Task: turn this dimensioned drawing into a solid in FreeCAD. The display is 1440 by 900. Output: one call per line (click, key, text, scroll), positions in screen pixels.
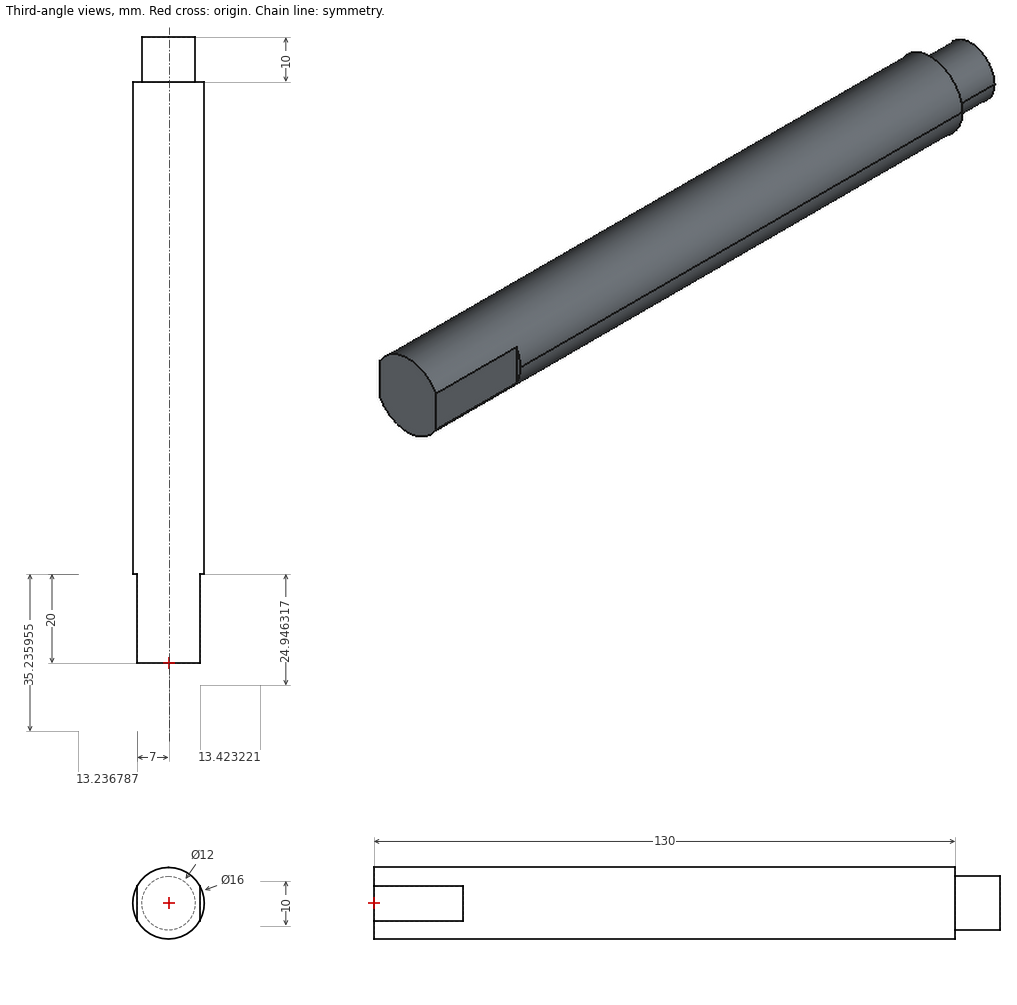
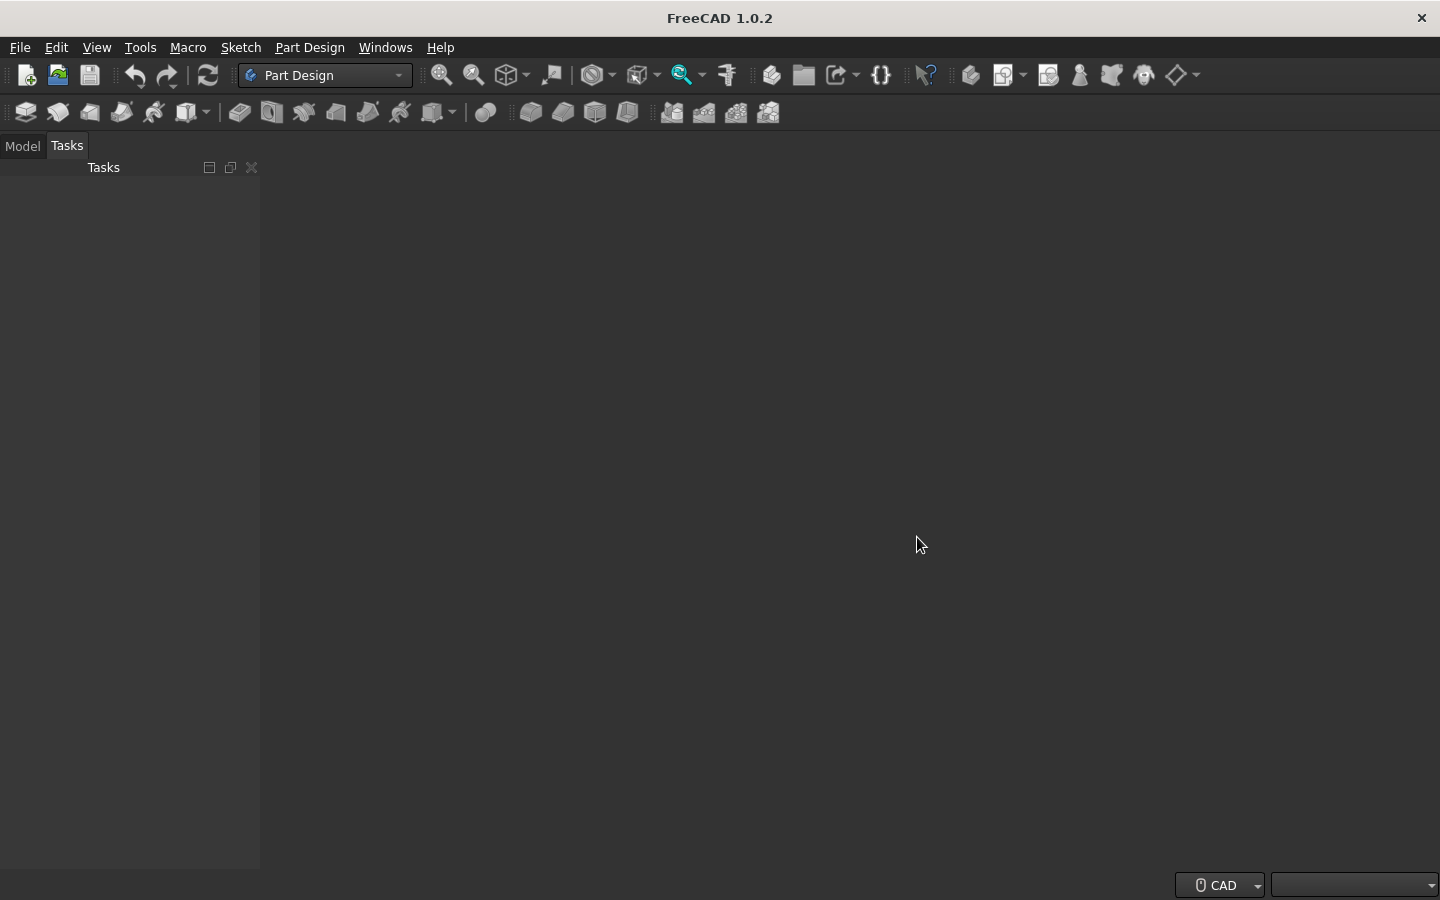
key(ctrl+n)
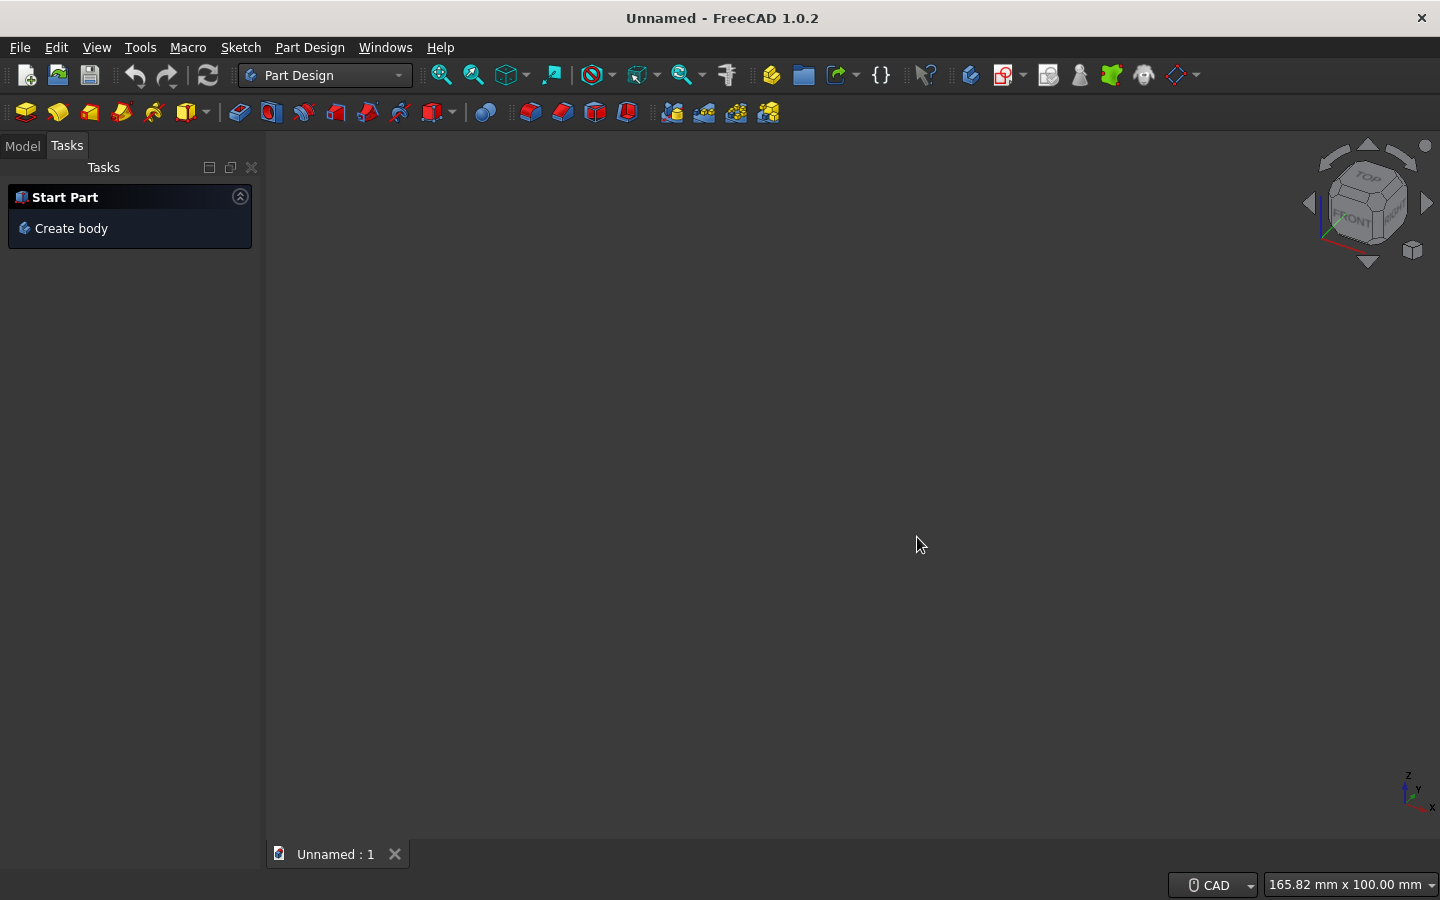
click(1004, 76)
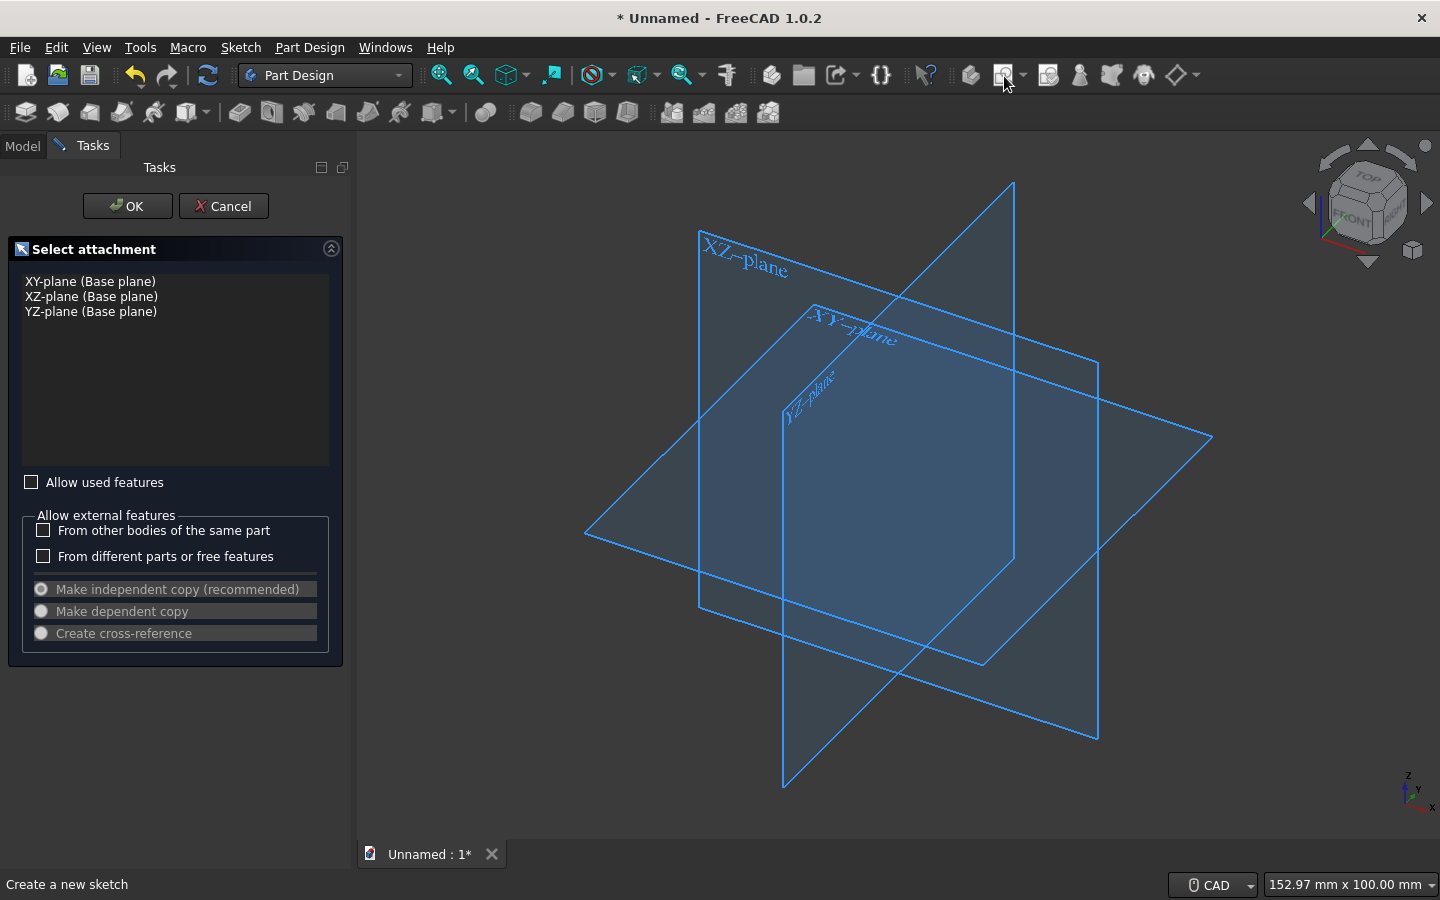
click(82, 296)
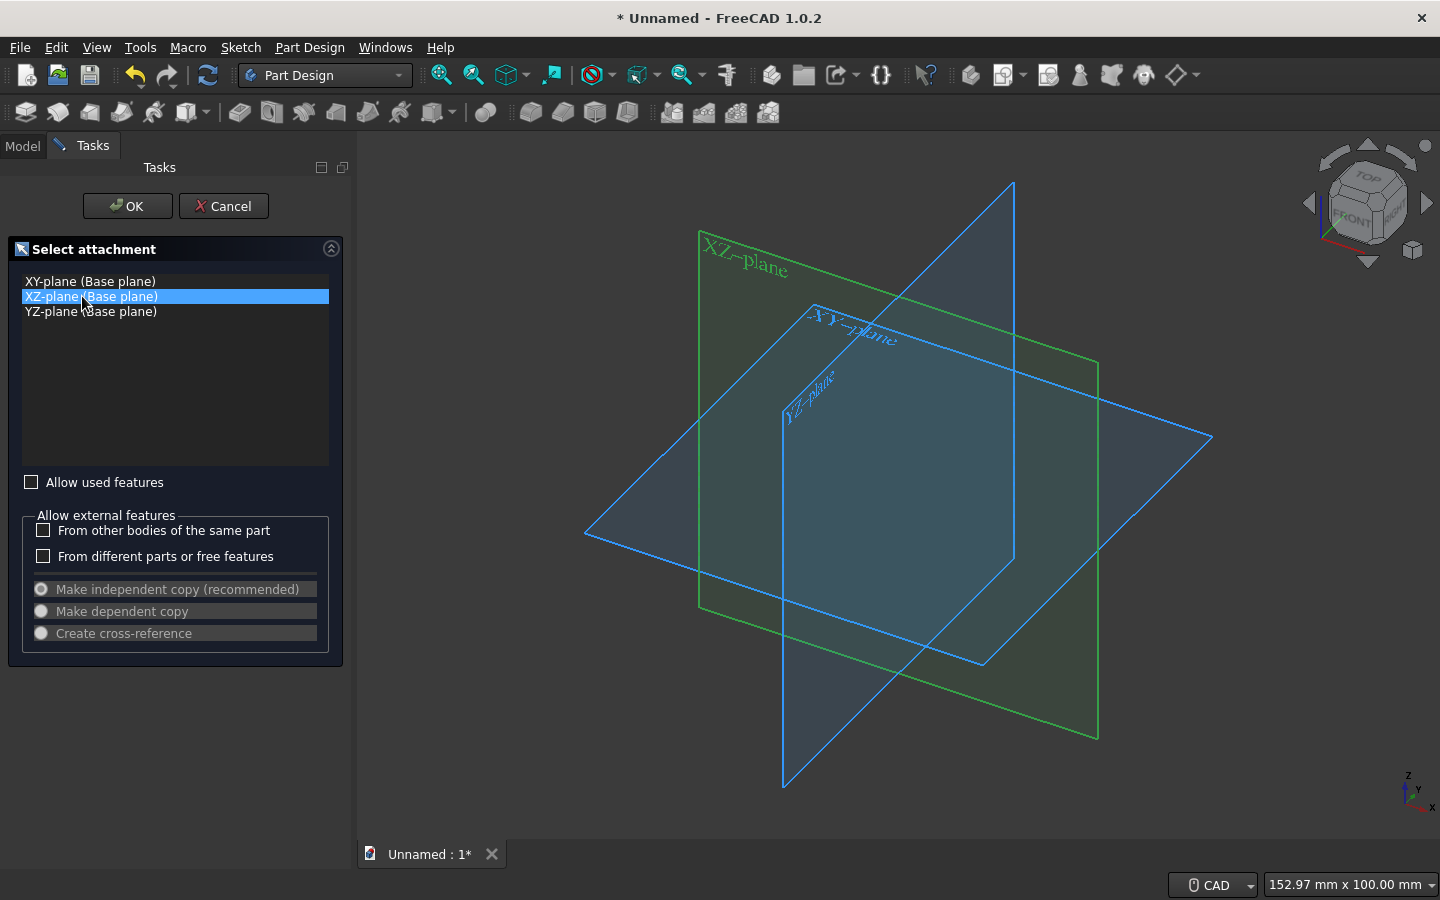
click(128, 206)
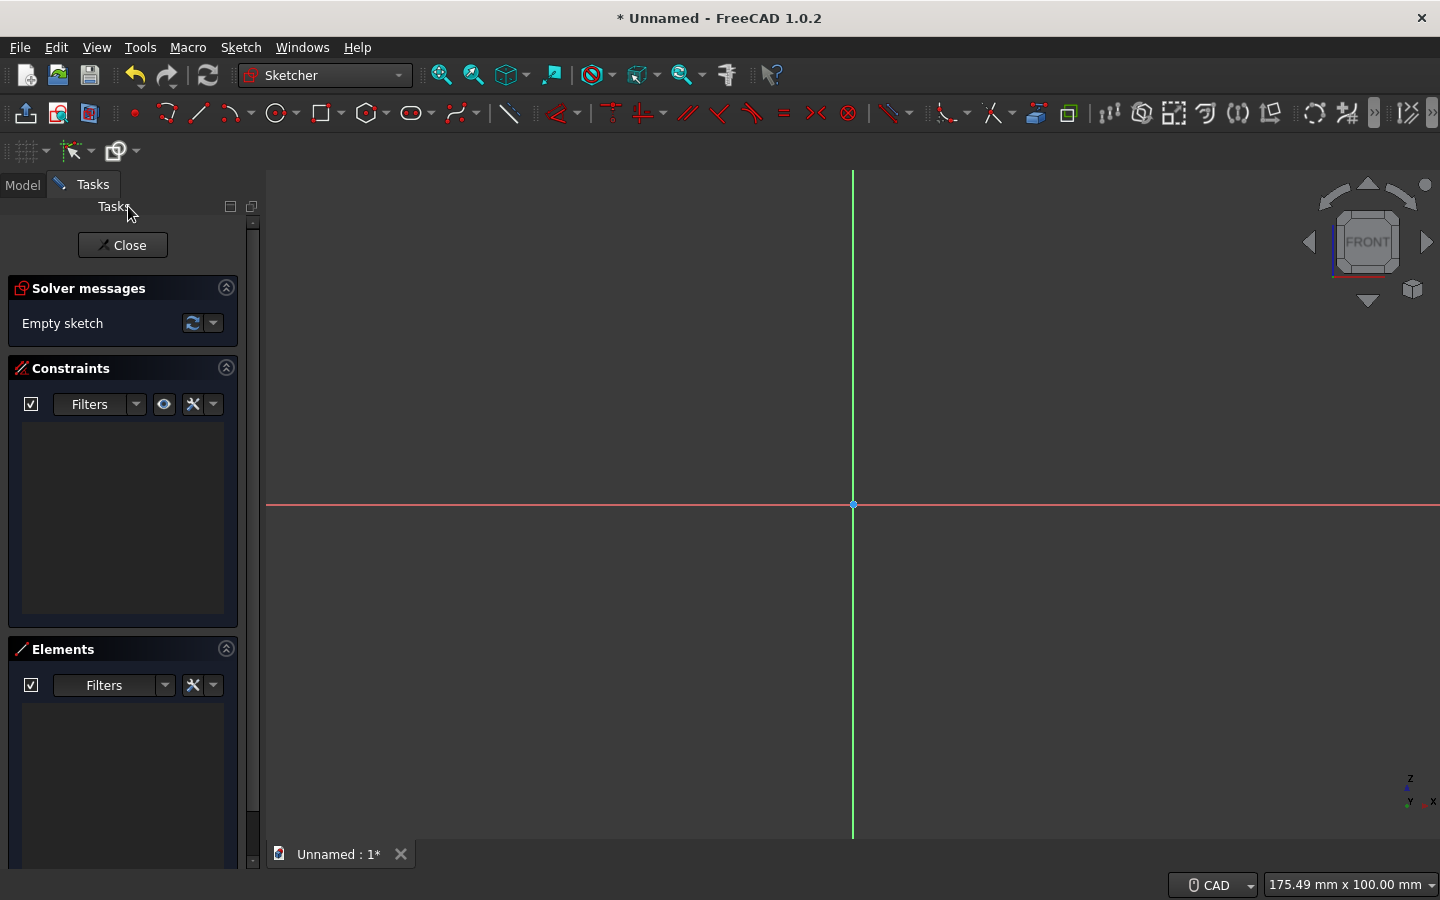
scroll(875, 504, up, 7)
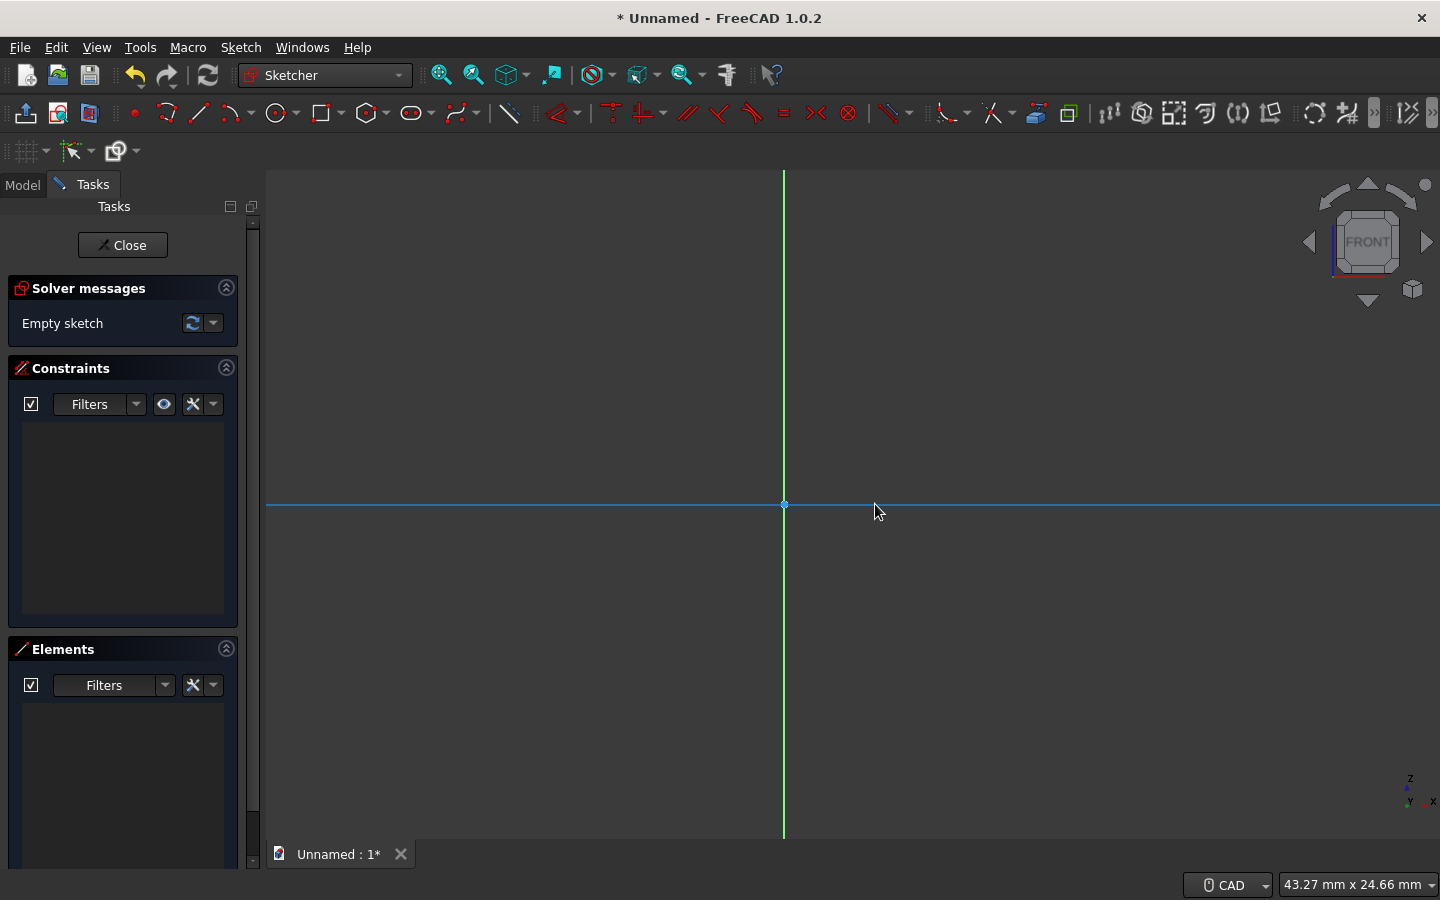
key(g)
key(c)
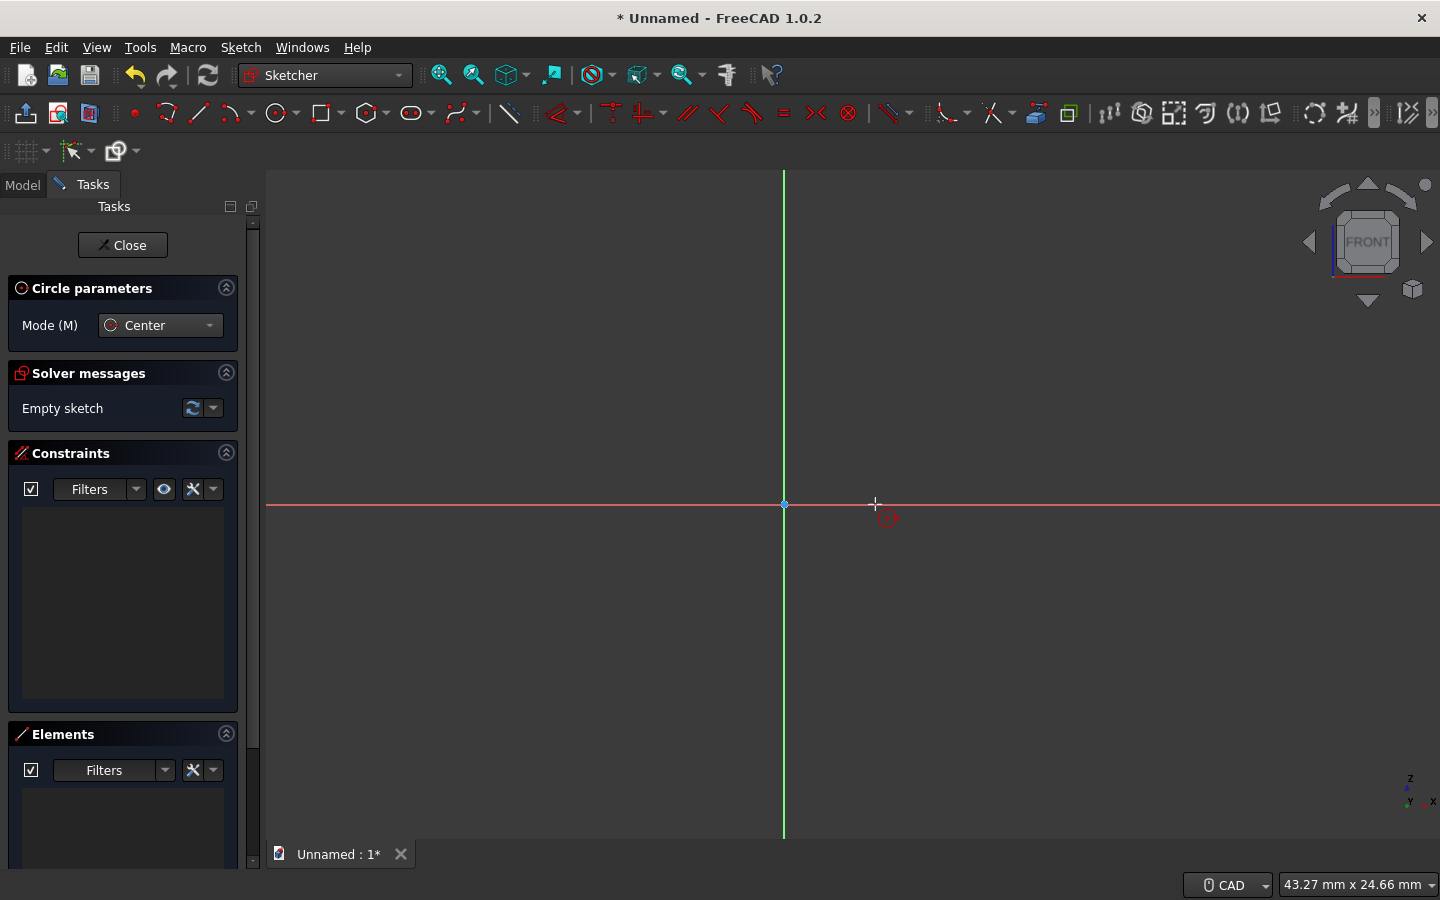
click(784, 504)
click(938, 351)
key(Escape)